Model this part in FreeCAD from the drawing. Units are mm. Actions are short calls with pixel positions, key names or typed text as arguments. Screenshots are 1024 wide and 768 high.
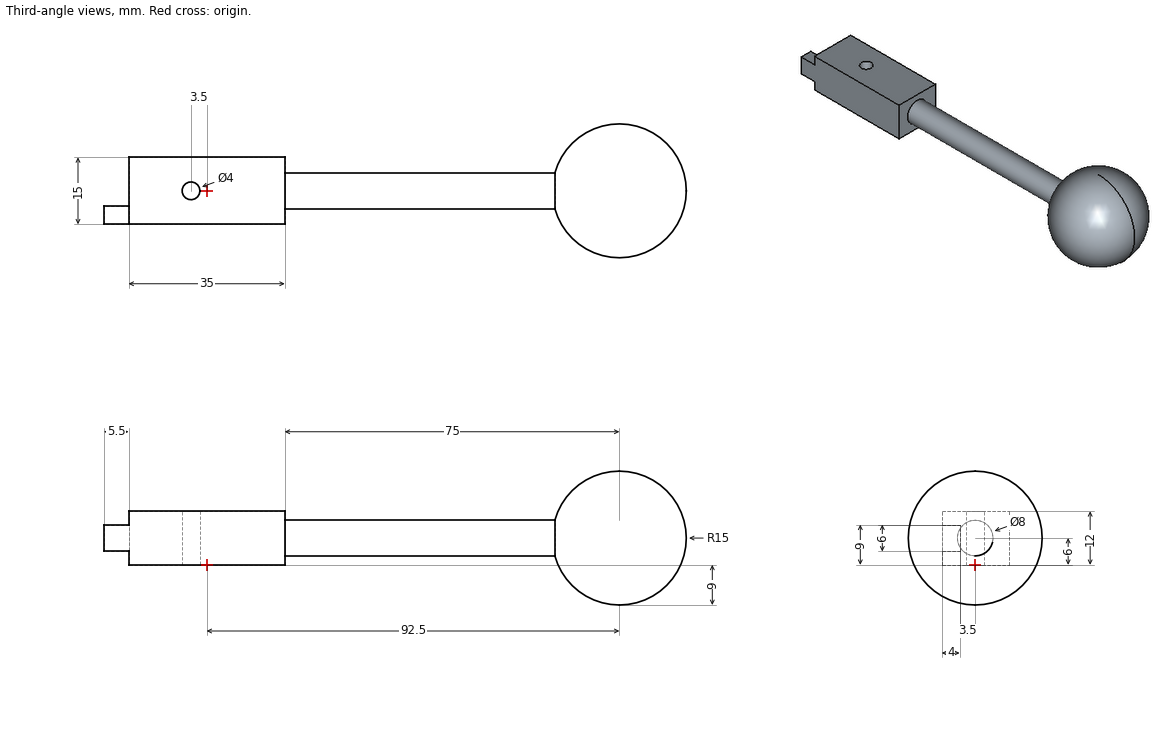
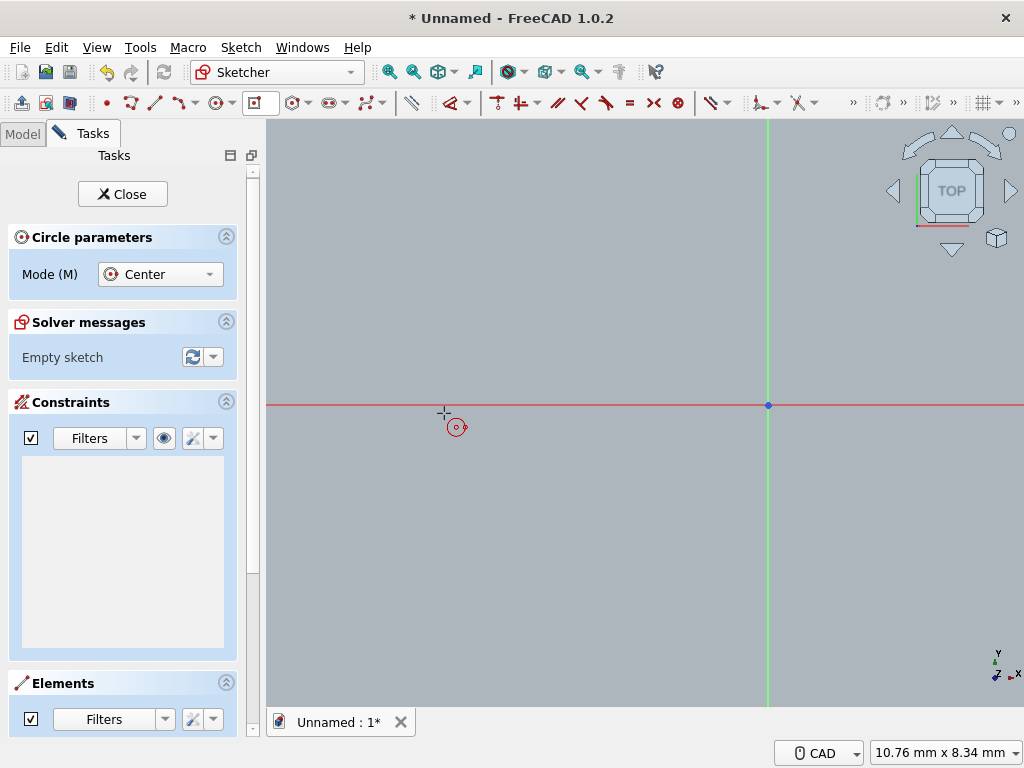
click(522, 405)
click(621, 306)
key(Escape)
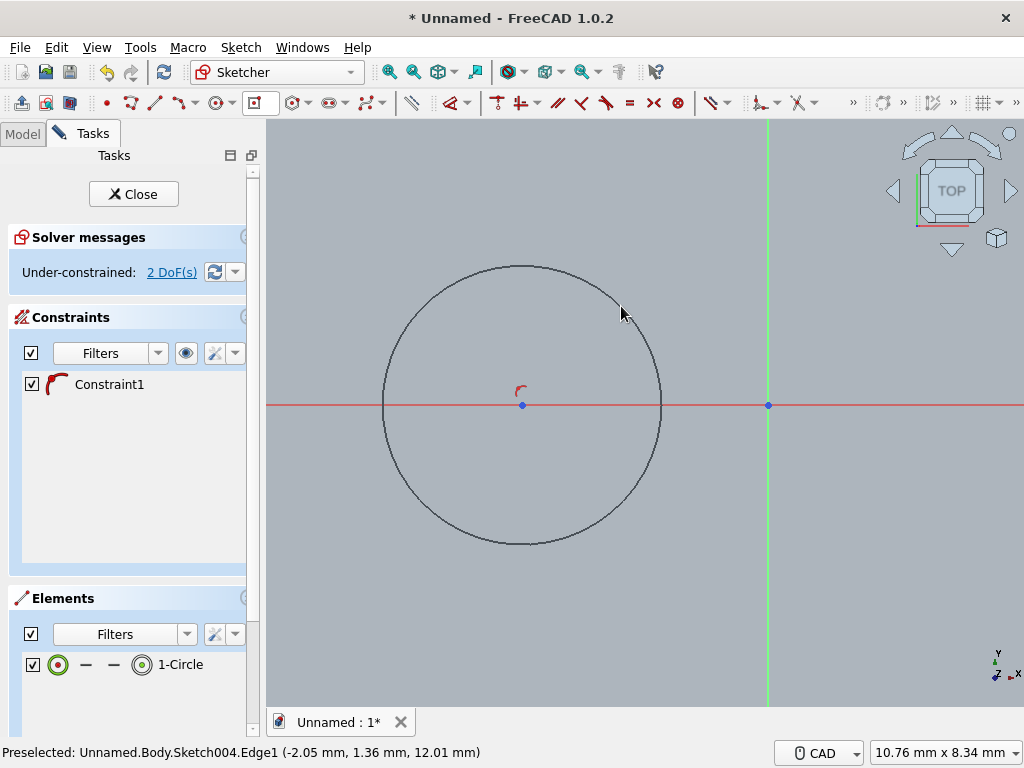
key(d)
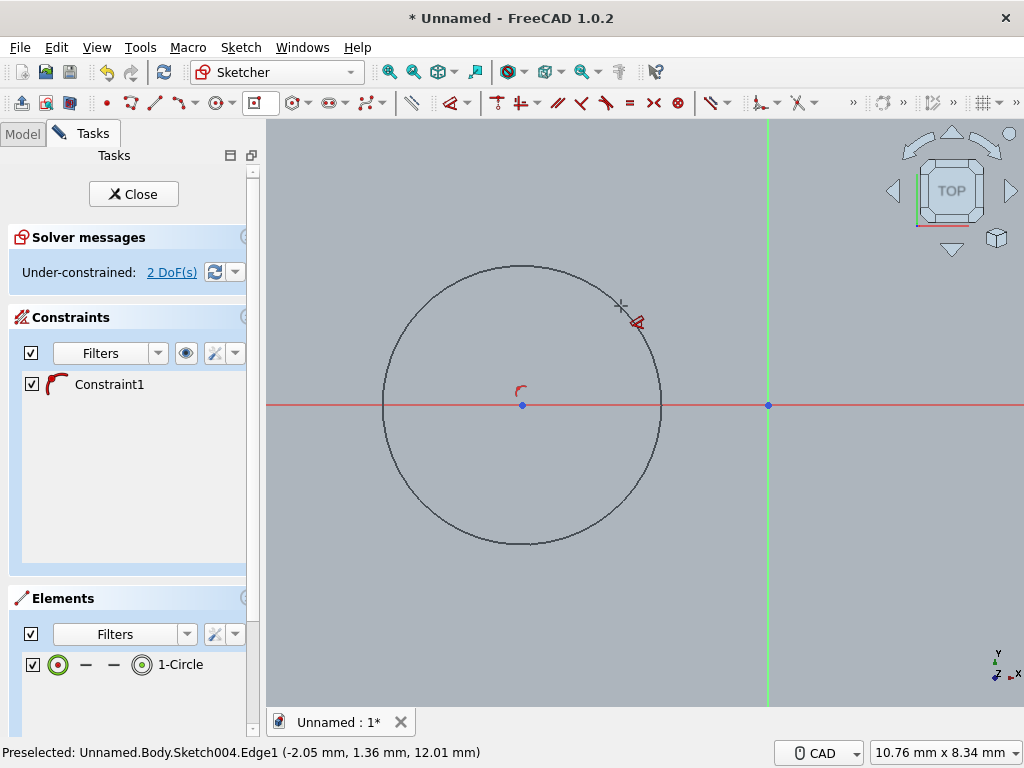
click(620, 306)
click(642, 283)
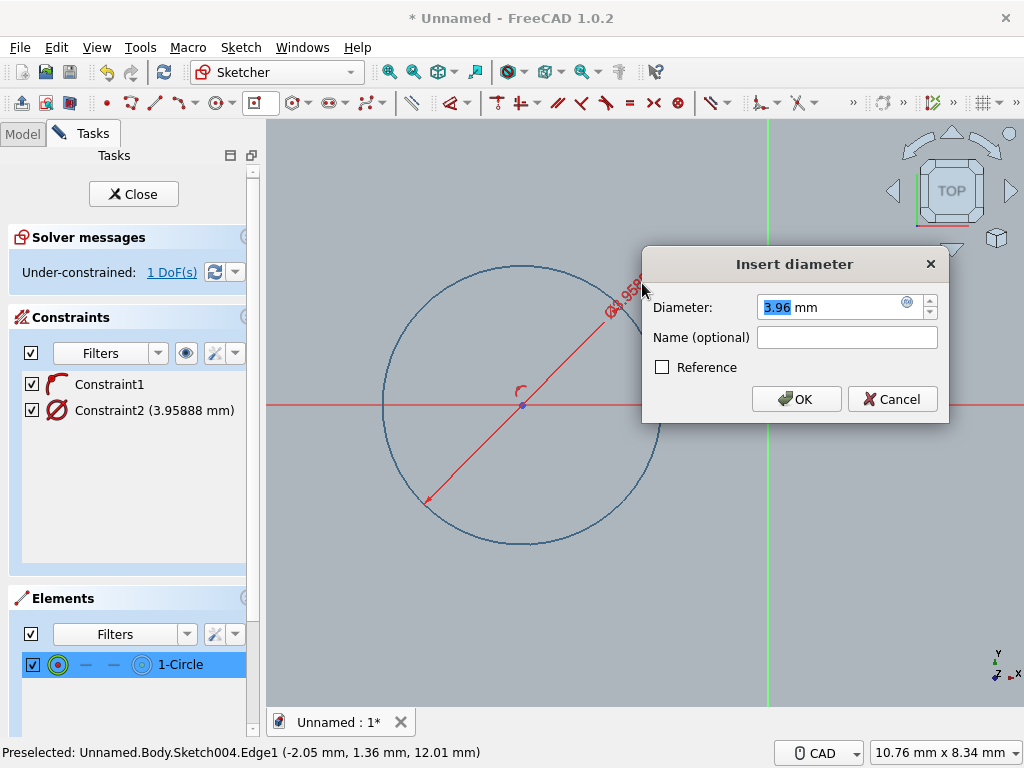
text(4)
key(Return)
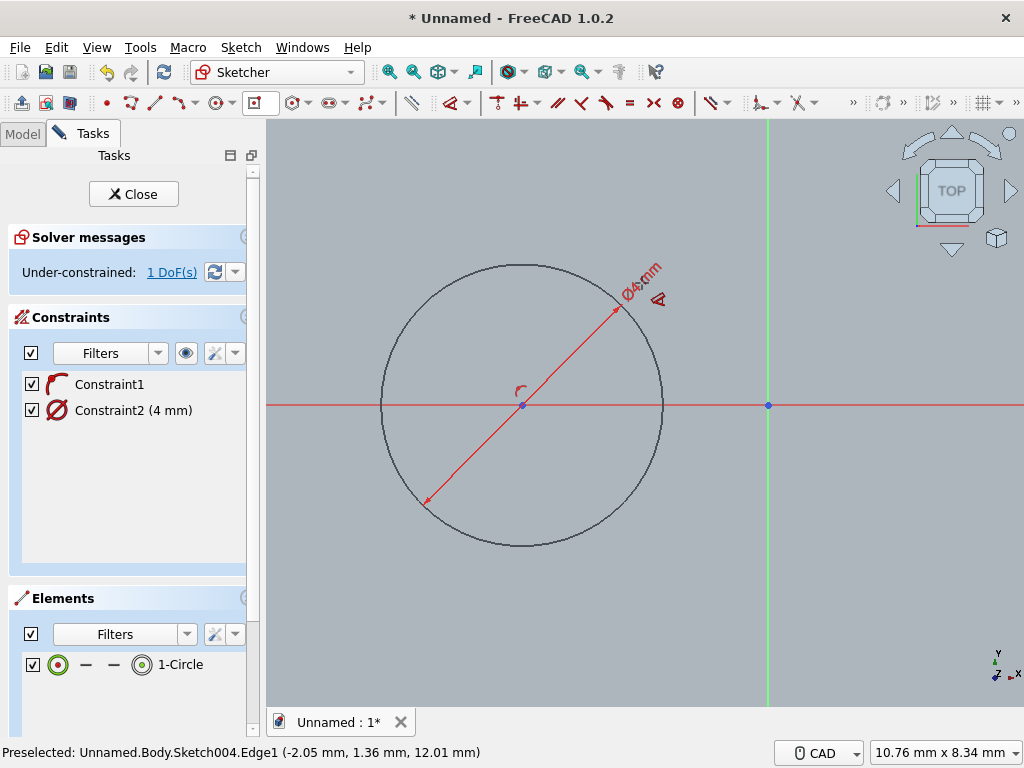
click(522, 405)
click(645, 439)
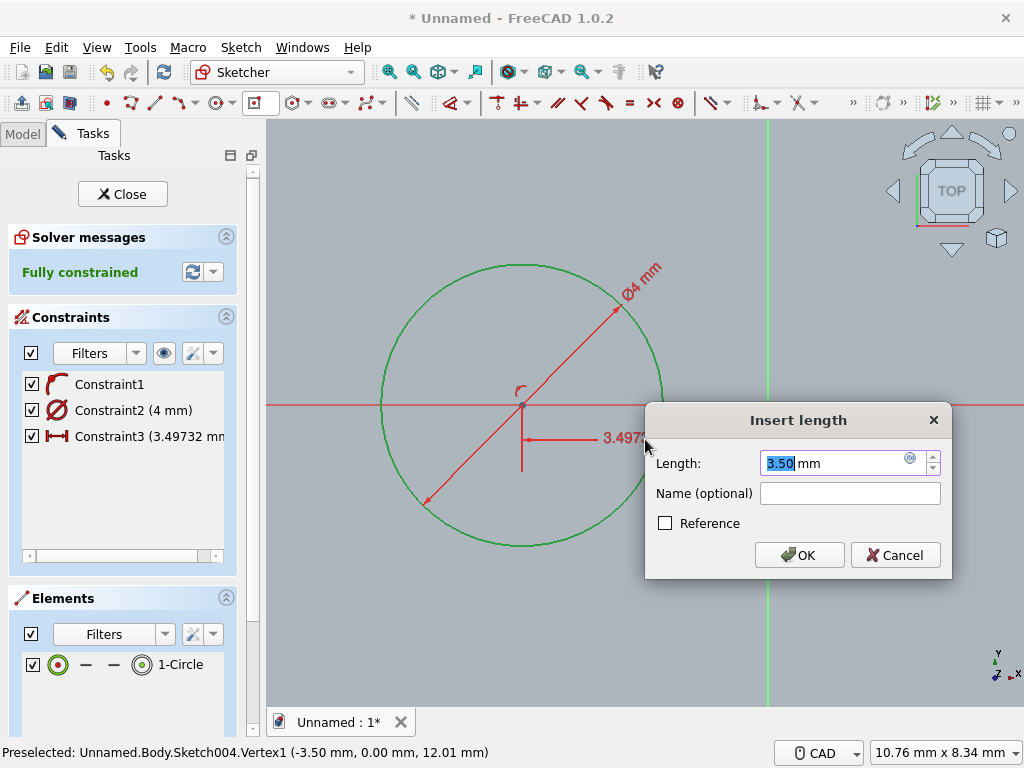
text(3.5)
key(Return)
key(Escape)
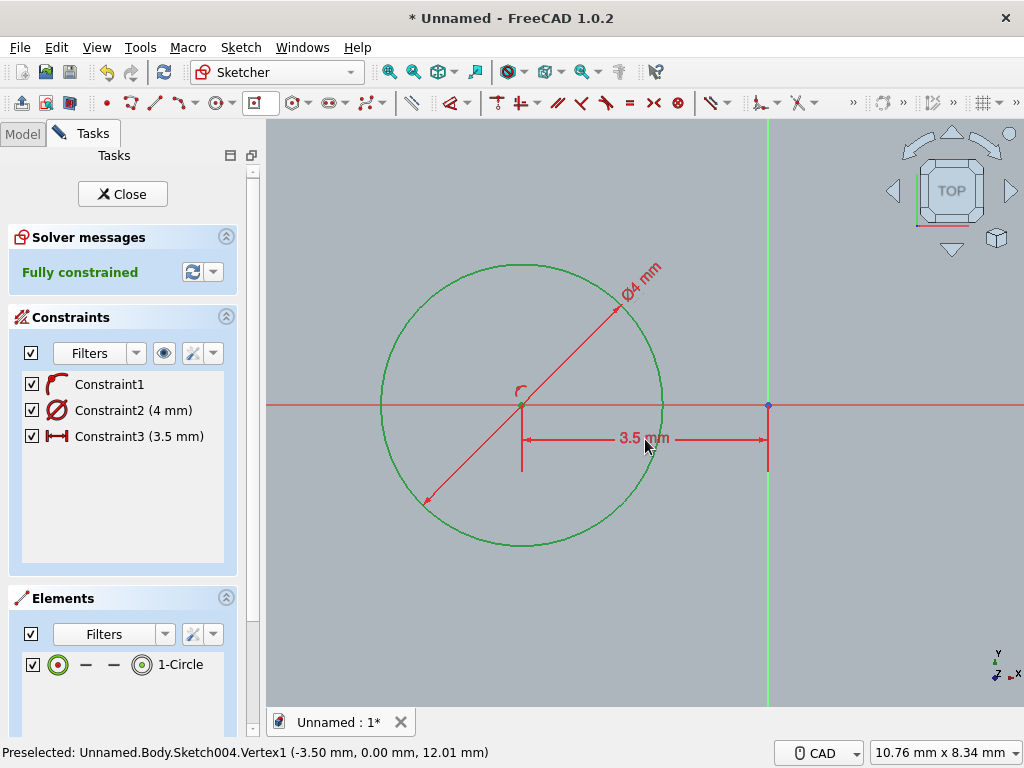
click(123, 194)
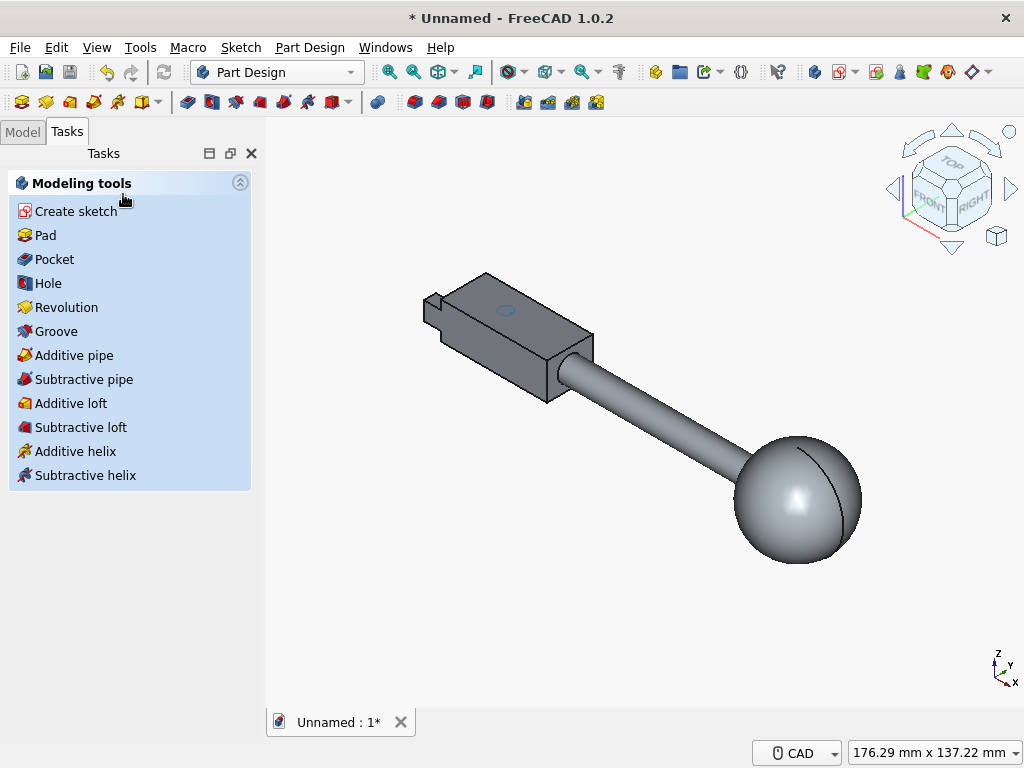
click(188, 102)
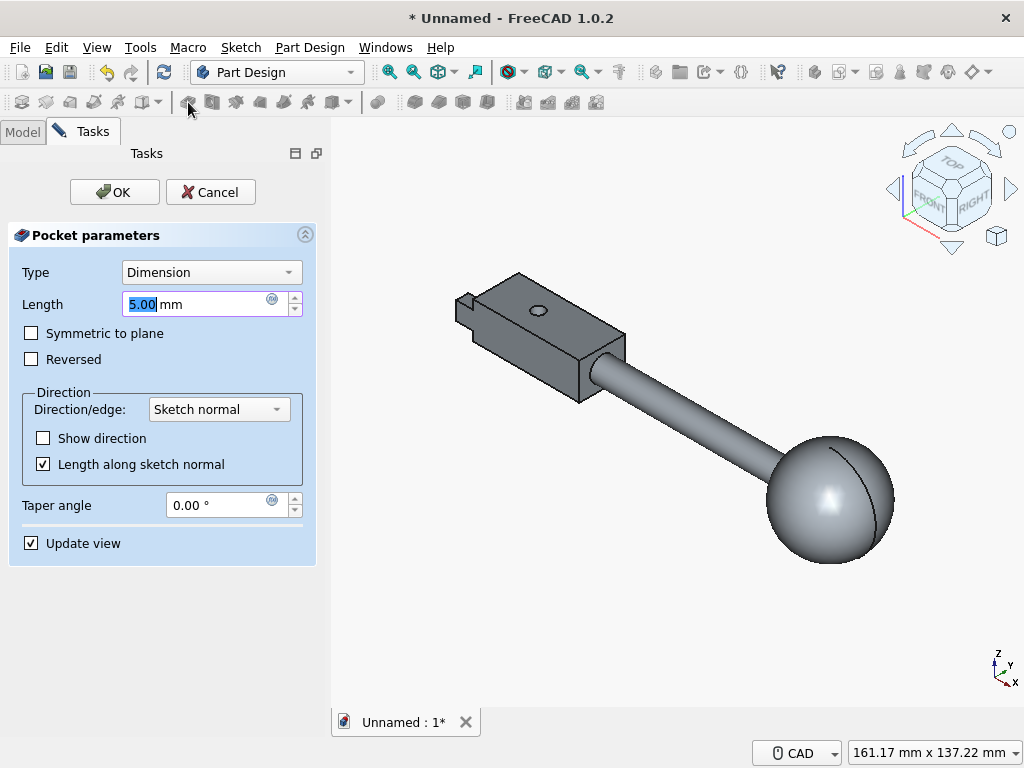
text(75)
key(Tab)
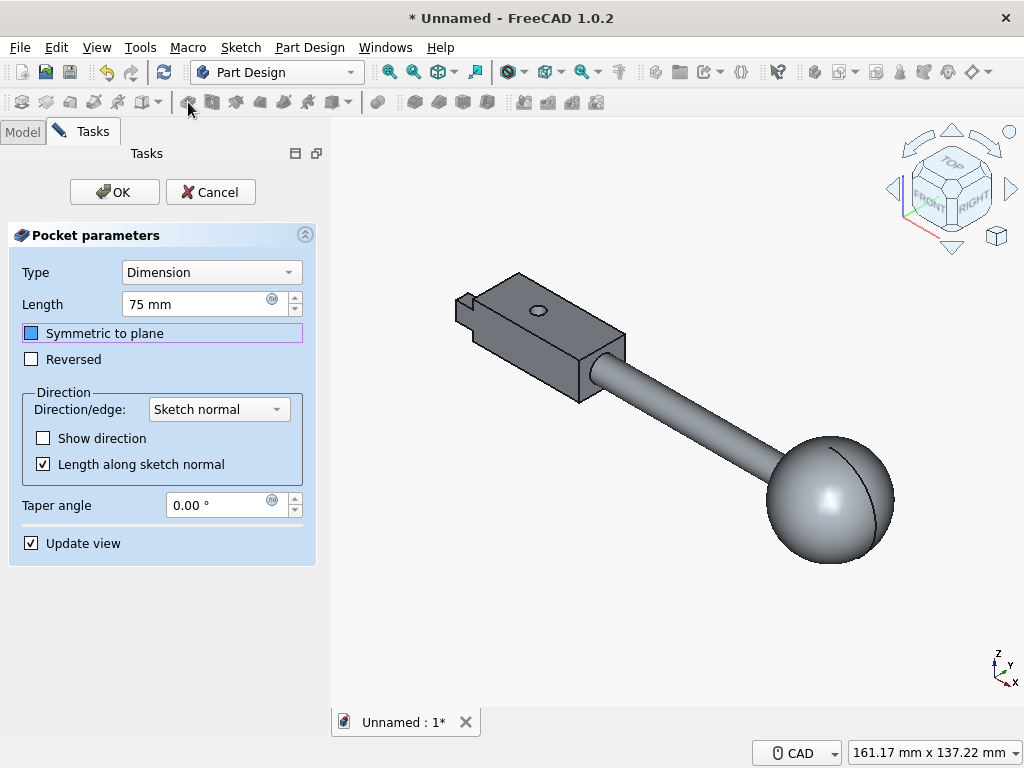
click(115, 192)